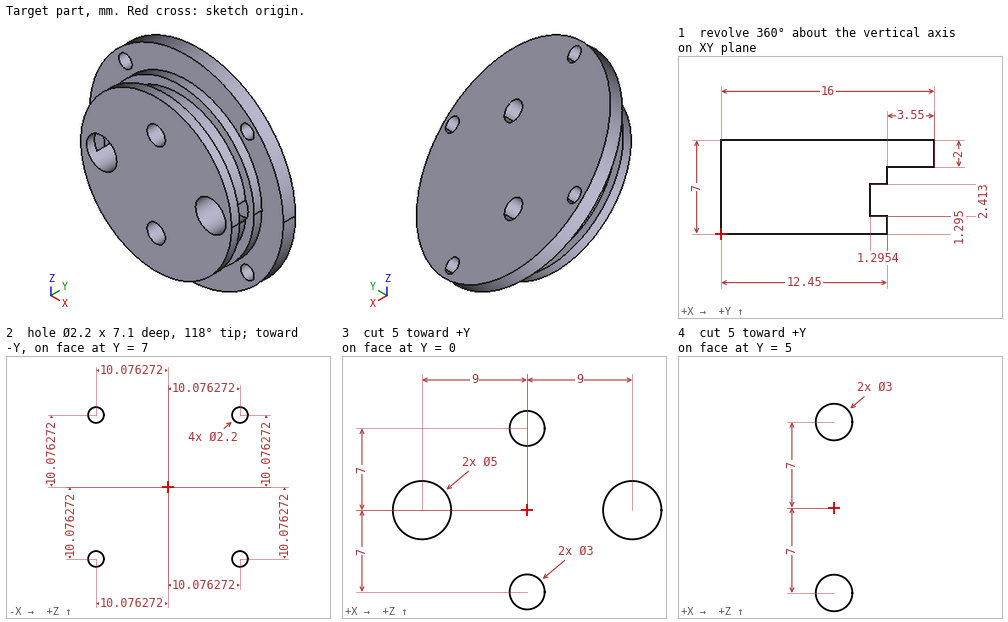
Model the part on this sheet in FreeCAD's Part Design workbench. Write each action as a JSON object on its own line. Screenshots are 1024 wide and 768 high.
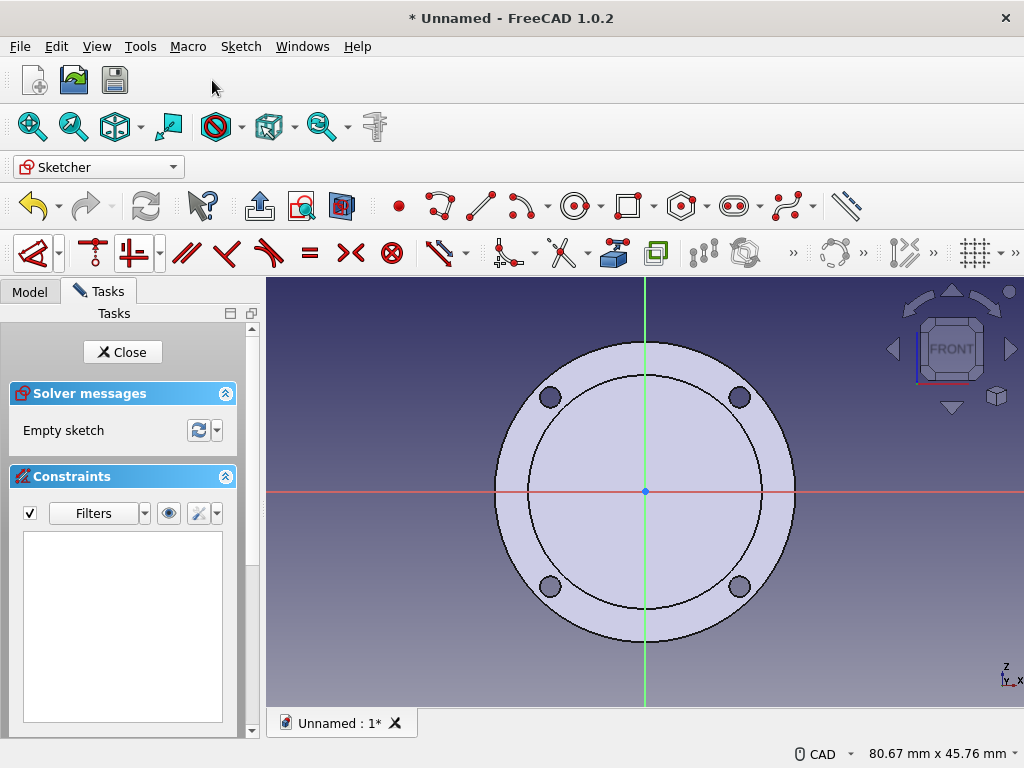
{"action": "scroll", "coordinate": [728, 492], "scroll_direction": "up", "scroll_amount": 3}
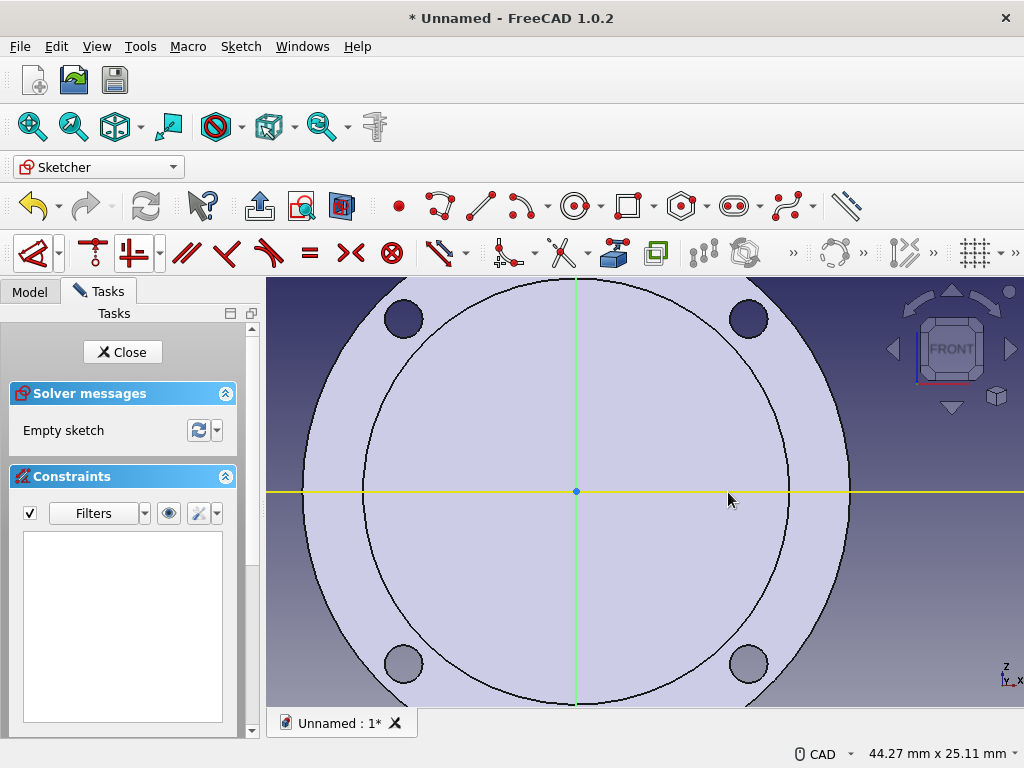
{"action": "left_click", "coordinate": [574, 206]}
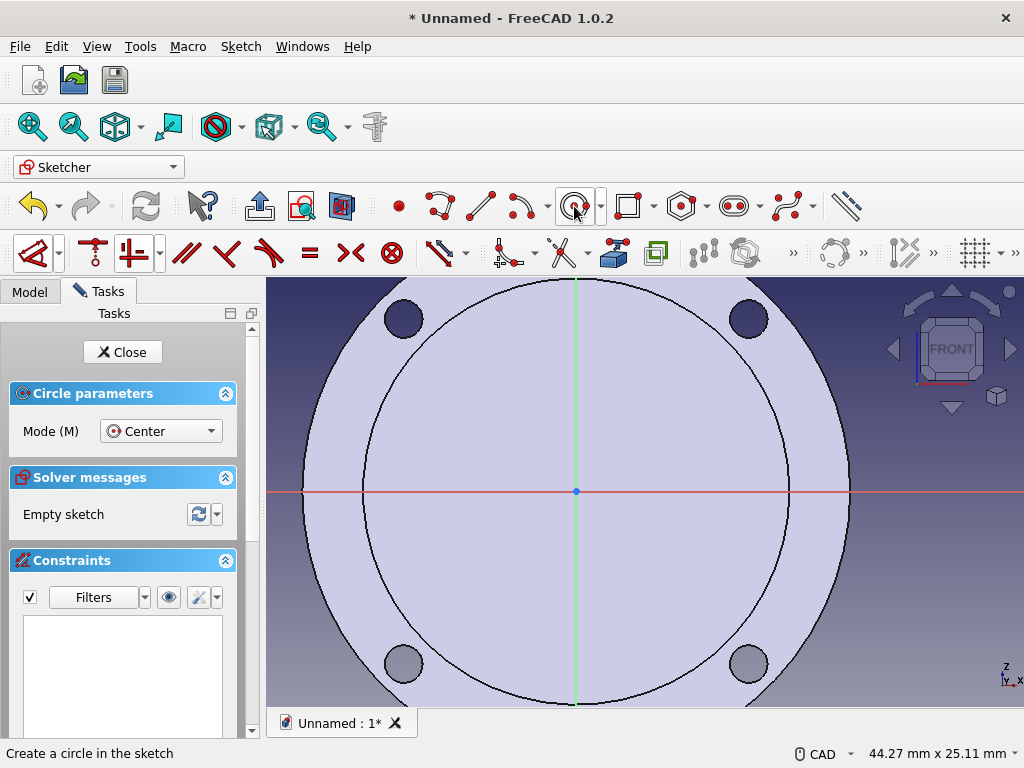
{"action": "left_click", "coordinate": [422, 492]}
{"action": "mouse_move", "coordinate": [452, 461]}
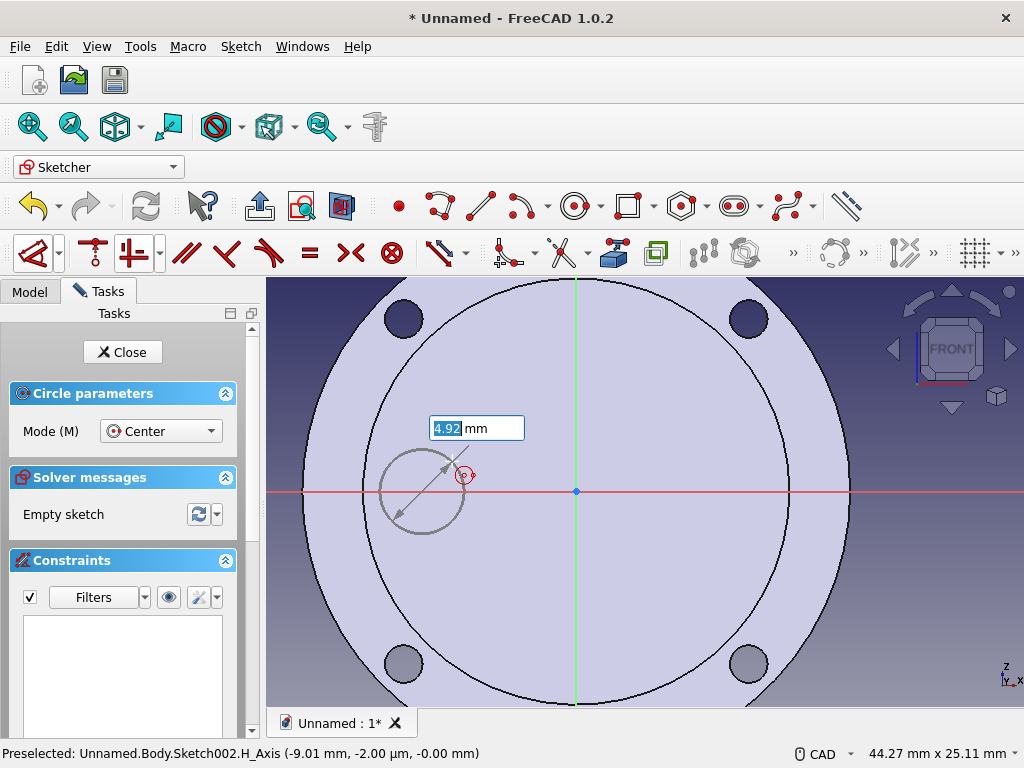
{"action": "type", "text": "5"}
{"action": "key", "text": "Return"}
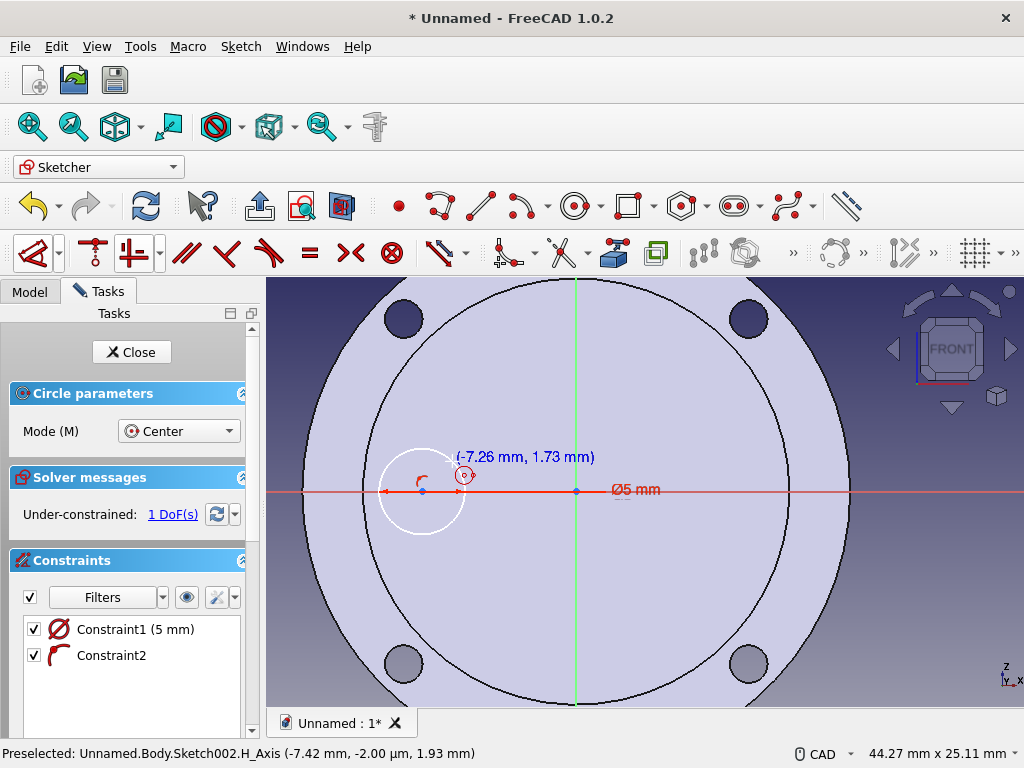
{"action": "left_click", "coordinate": [730, 492]}
{"action": "mouse_move", "coordinate": [761, 461]}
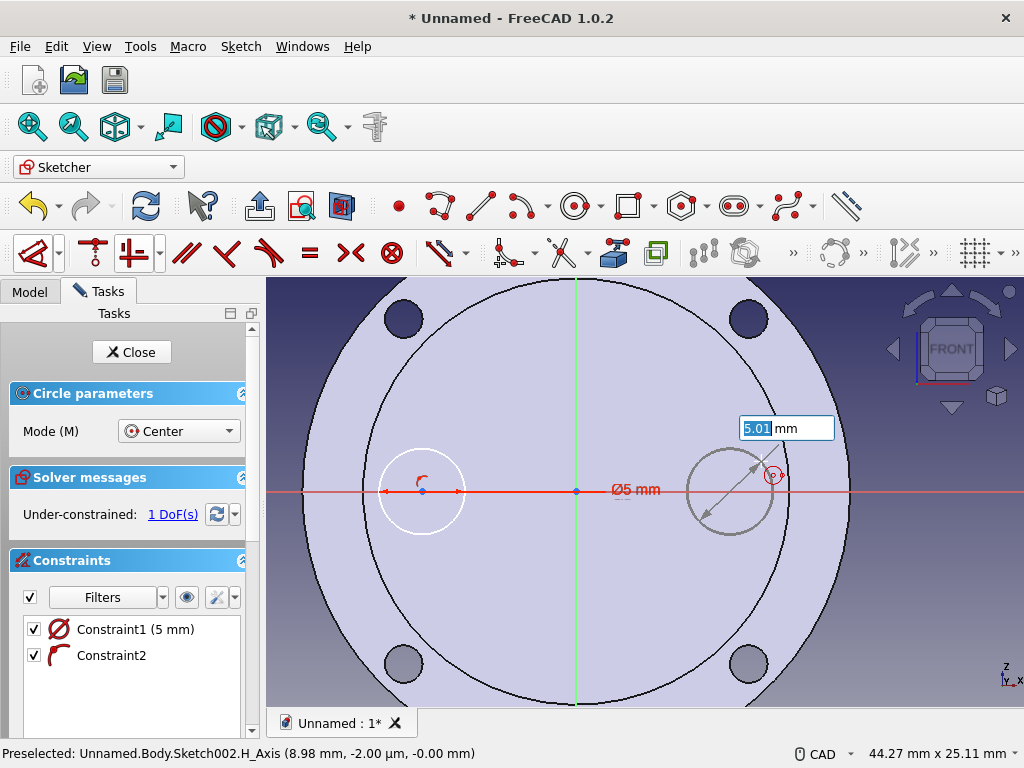
{"action": "type", "text": "5"}
{"action": "key", "text": "Return"}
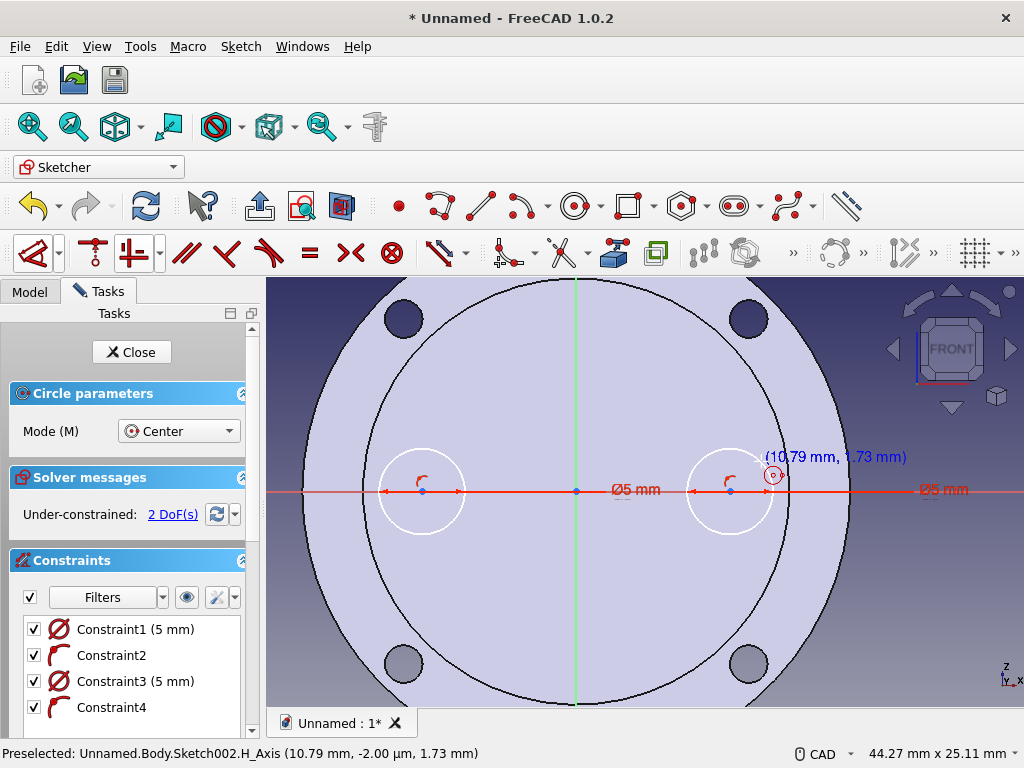
{"action": "left_click", "coordinate": [576, 611]}
{"action": "mouse_move", "coordinate": [594, 593]}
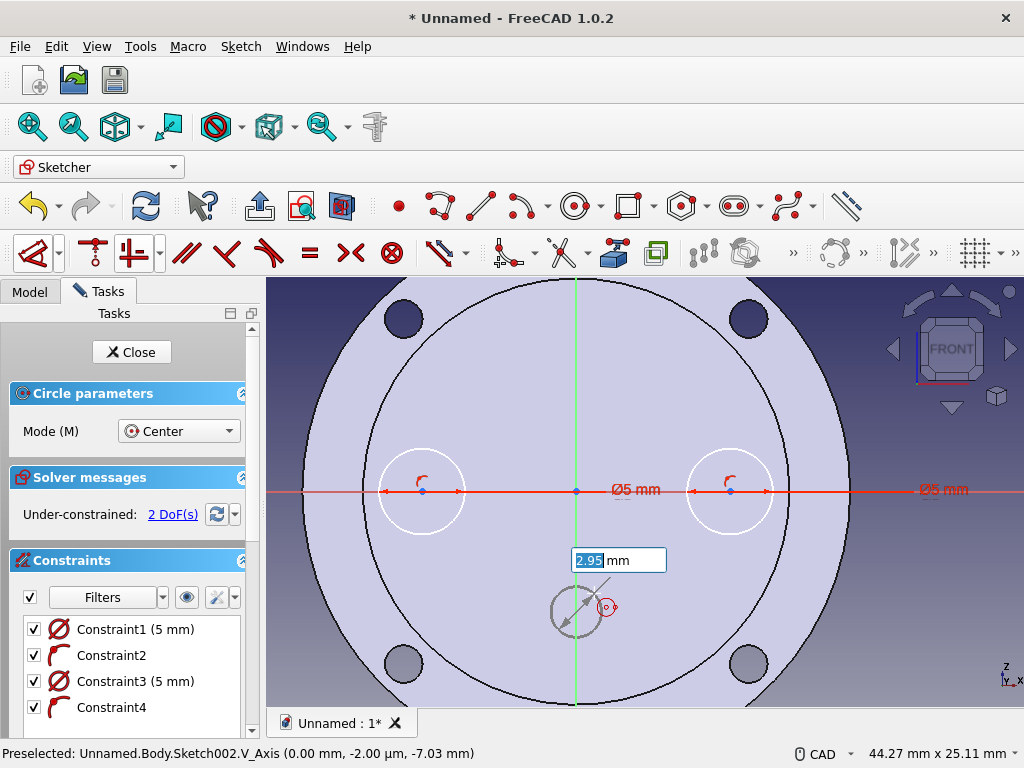
{"action": "type", "text": "3"}
{"action": "key", "text": "Return"}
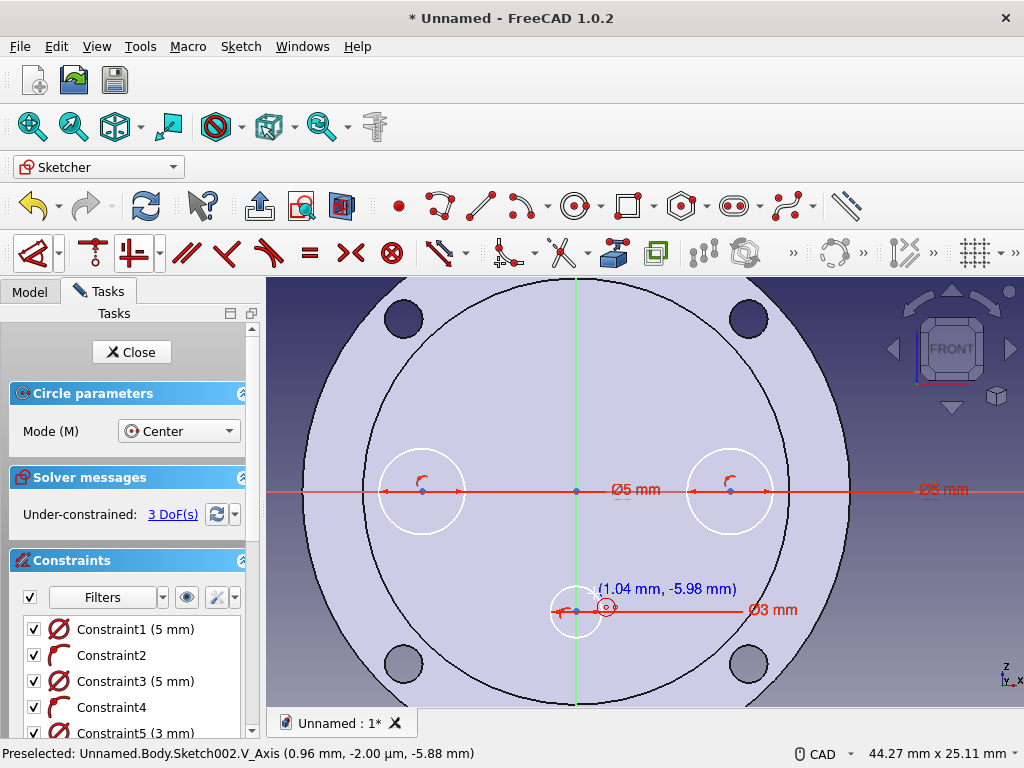
{"action": "left_click", "coordinate": [576, 372]}
{"action": "mouse_move", "coordinate": [594, 354]}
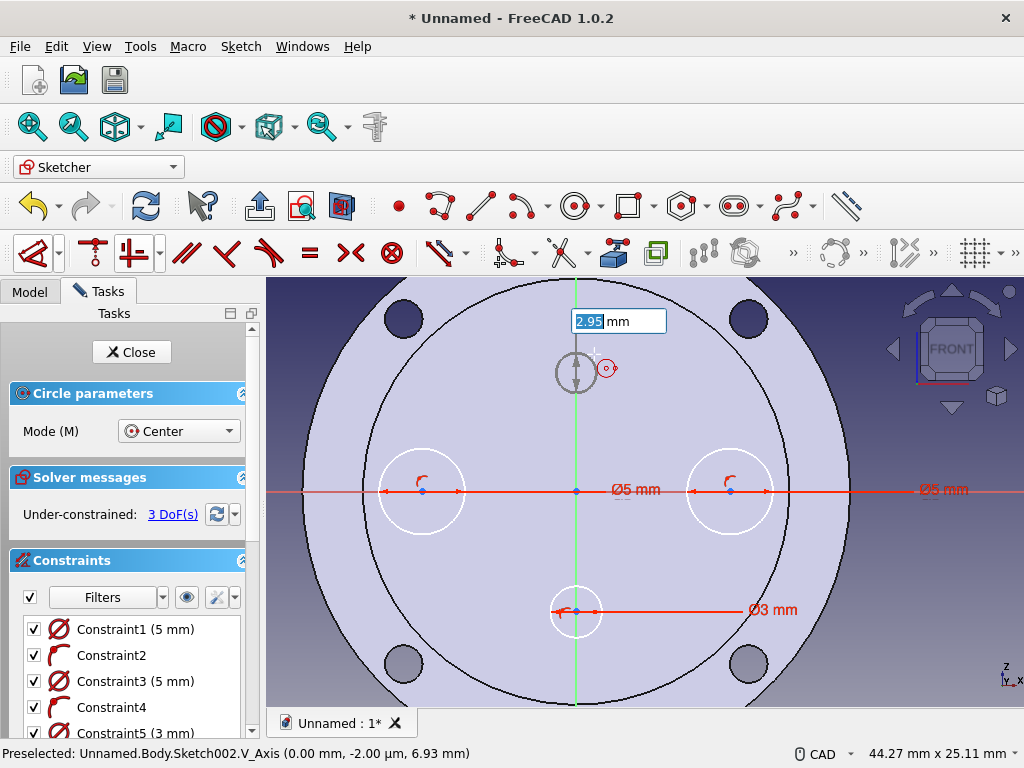
{"action": "type", "text": "3"}
{"action": "key", "text": "Return"}
{"action": "key", "text": "Escape"}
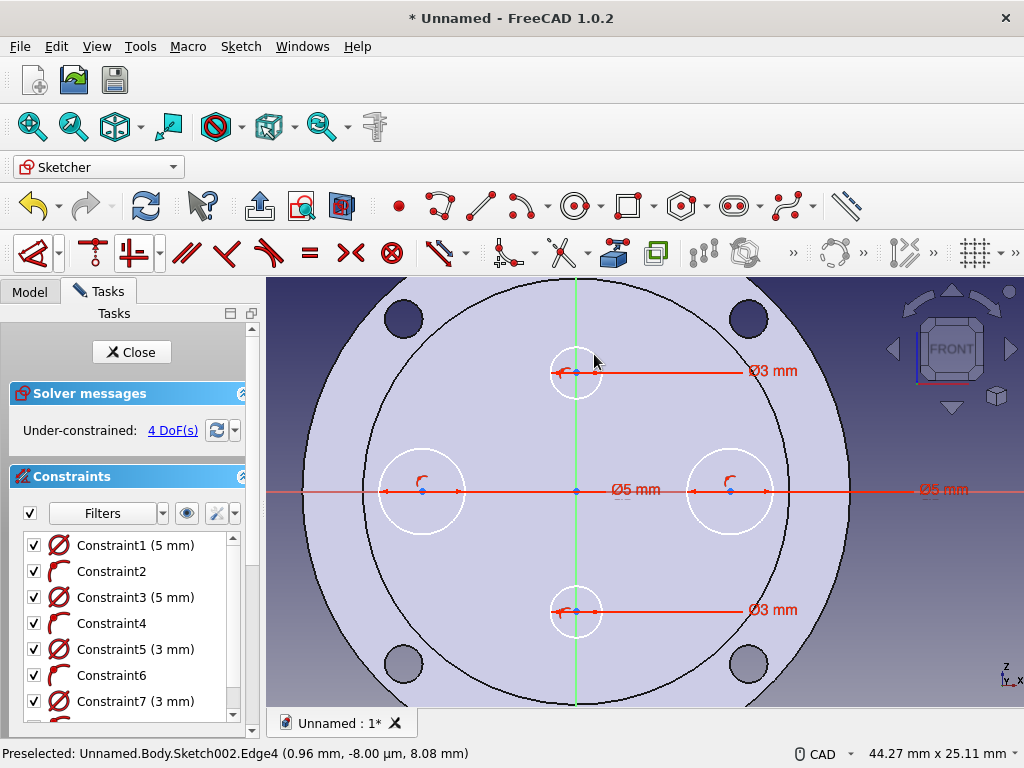
{"action": "left_click", "coordinate": [422, 492]}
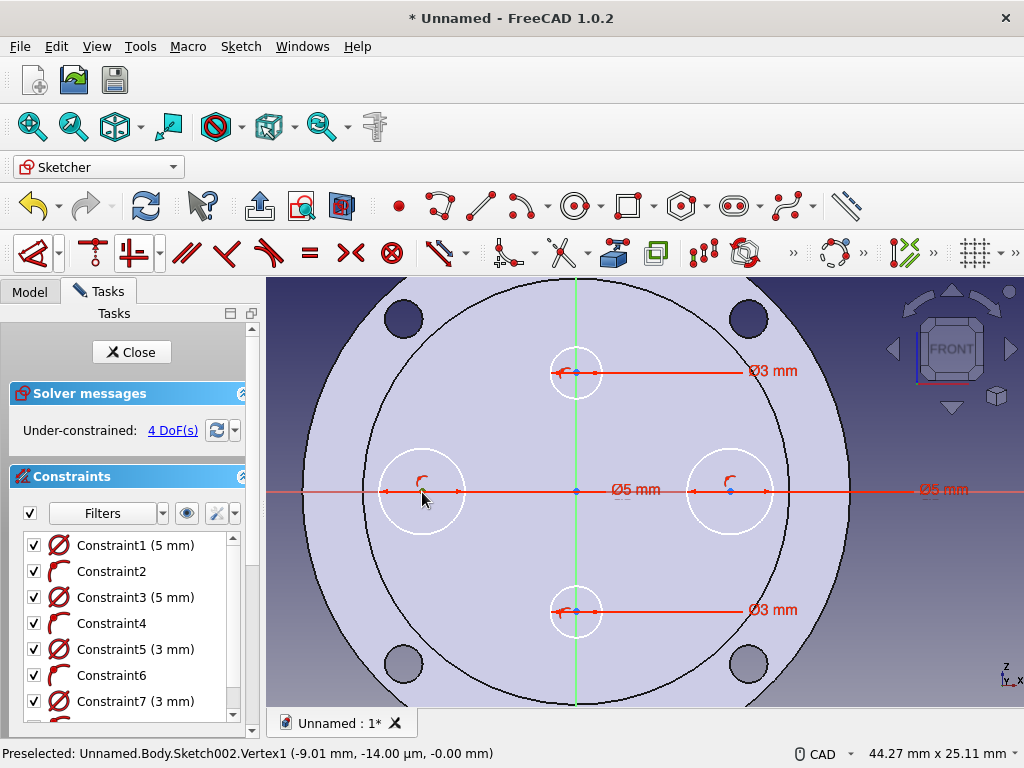
{"action": "left_click", "coordinate": [58, 254]}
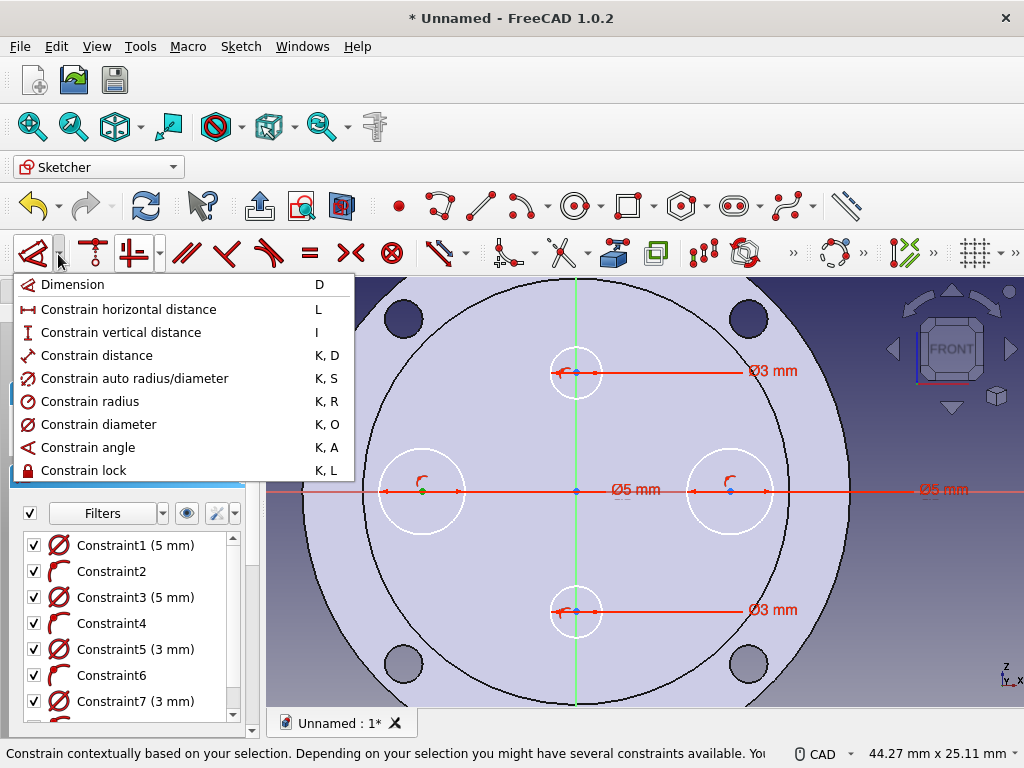
{"action": "left_click", "coordinate": [184, 310]}